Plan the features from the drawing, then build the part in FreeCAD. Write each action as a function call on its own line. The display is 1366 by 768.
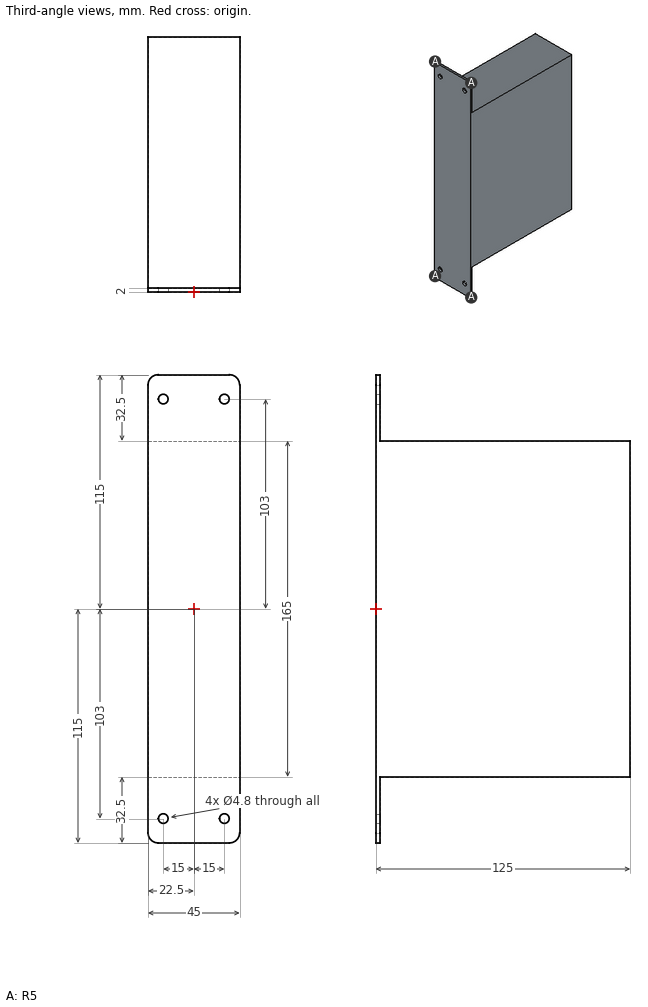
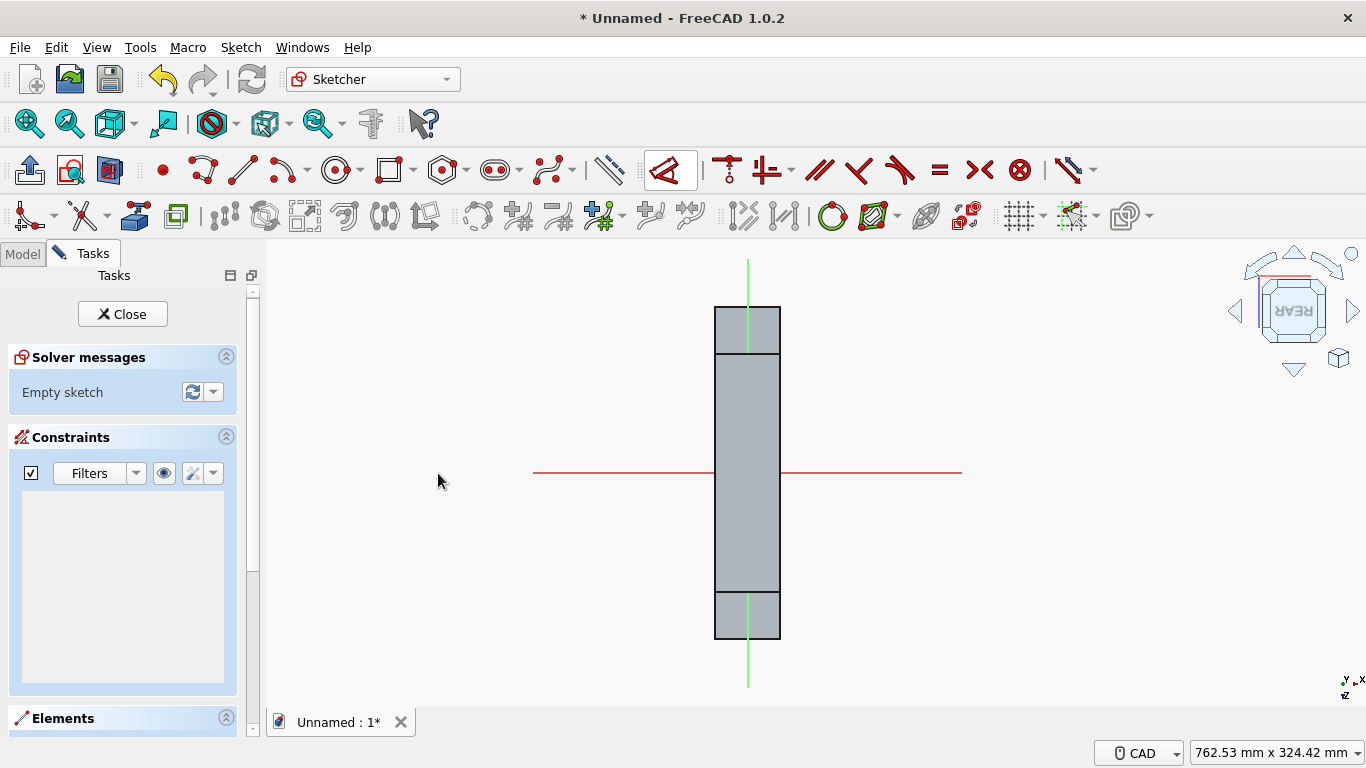
click(336, 170)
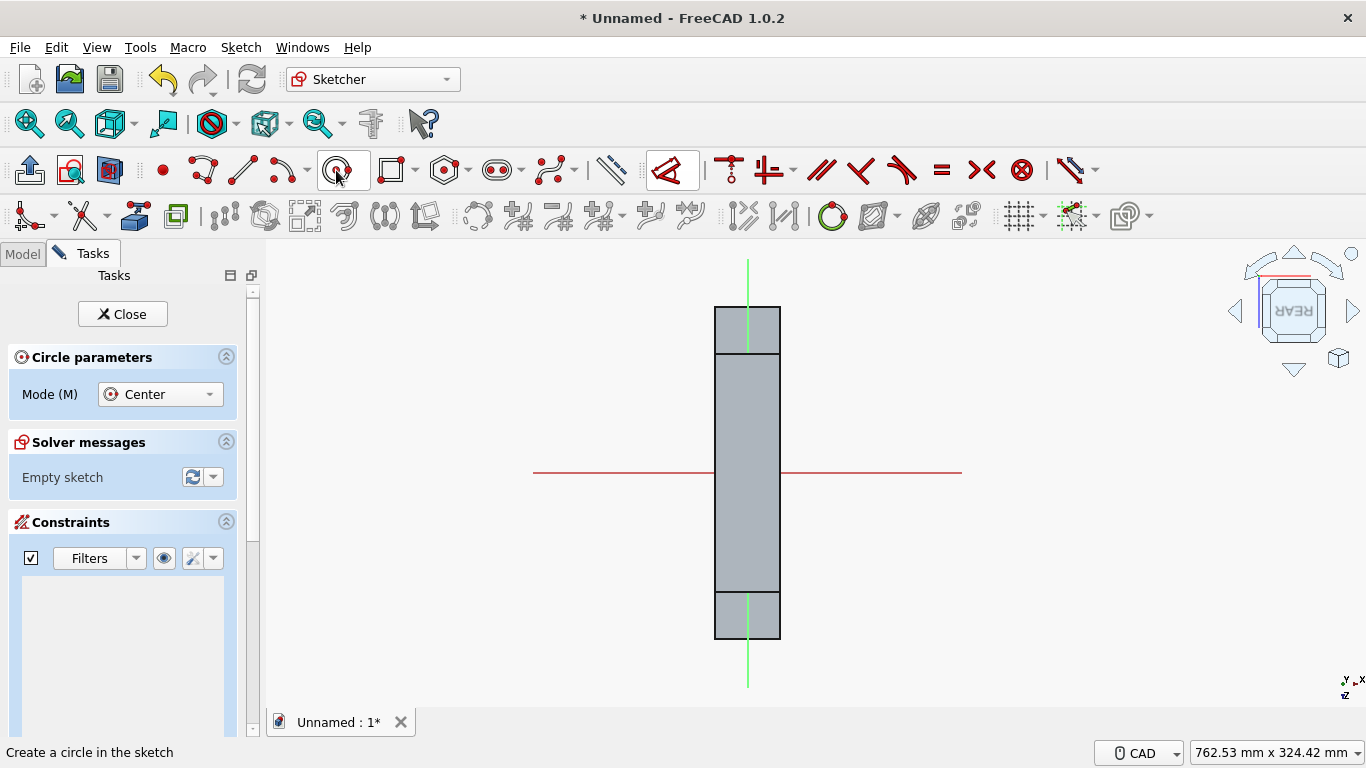
scroll(726, 325, up, 10)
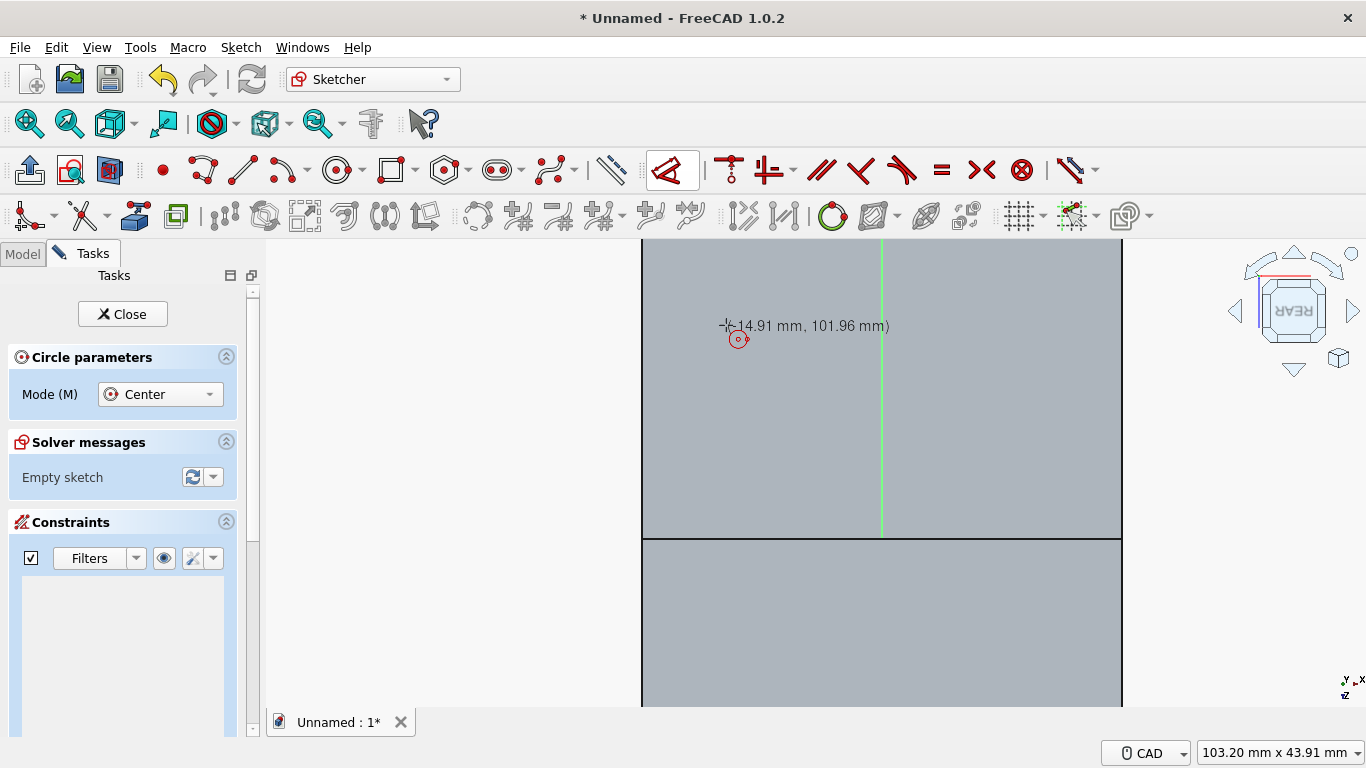
scroll(726, 325, down, 10)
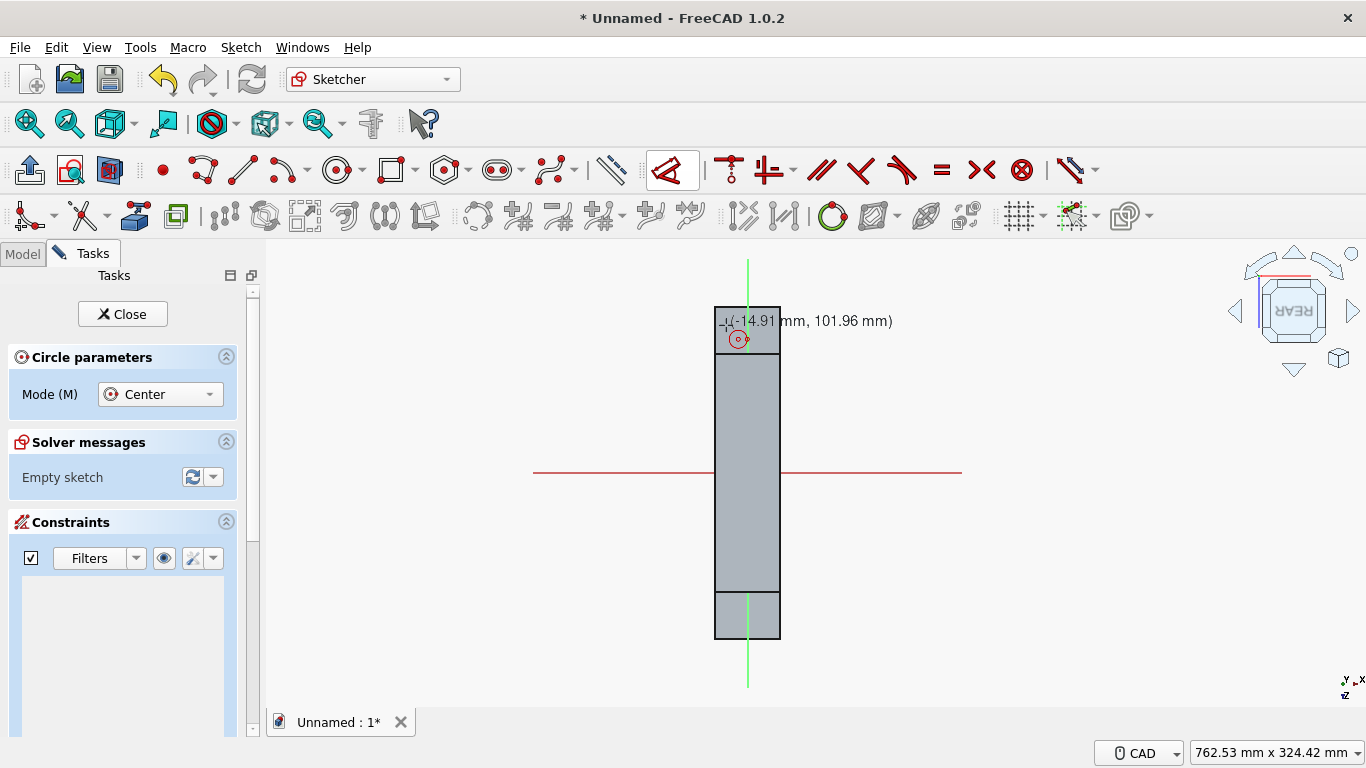
click(726, 325)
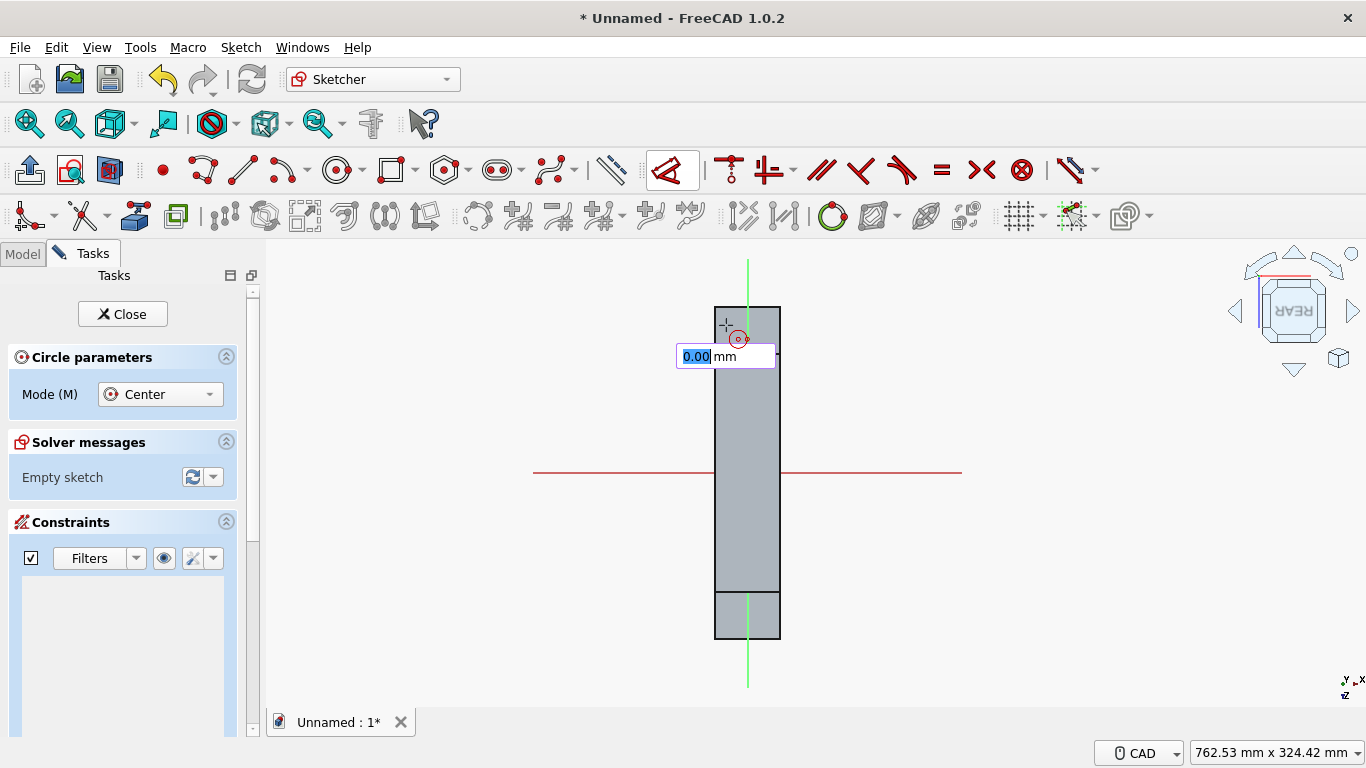
scroll(728, 322, up, 8)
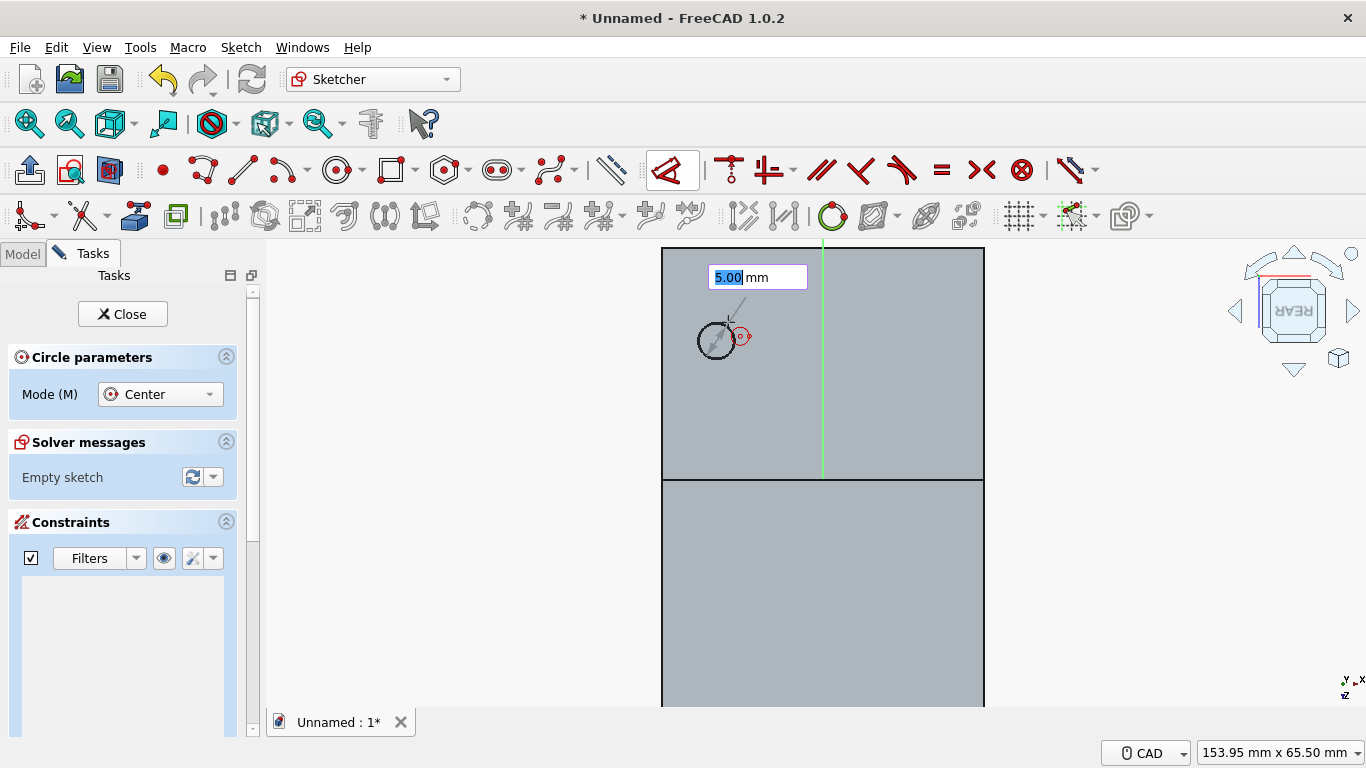
click(728, 322)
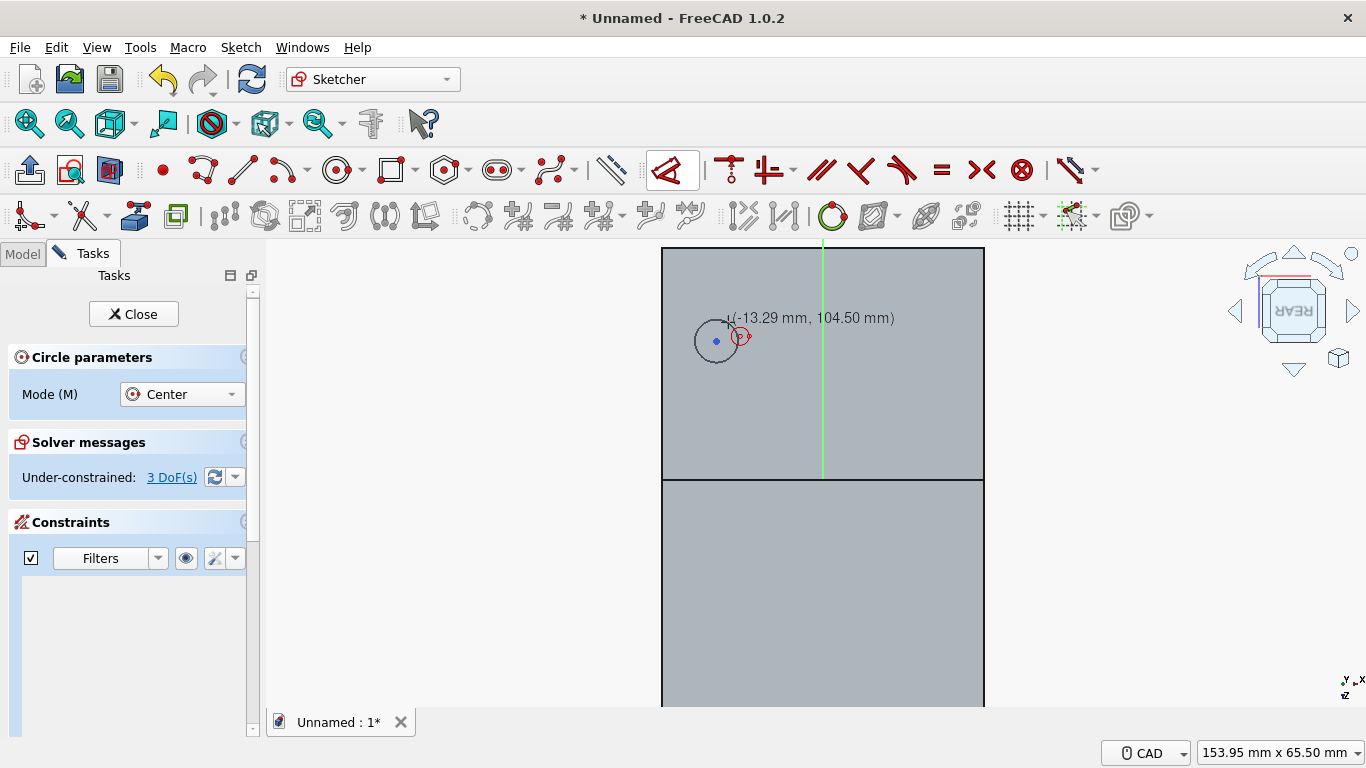
scroll(930, 334, up, 2)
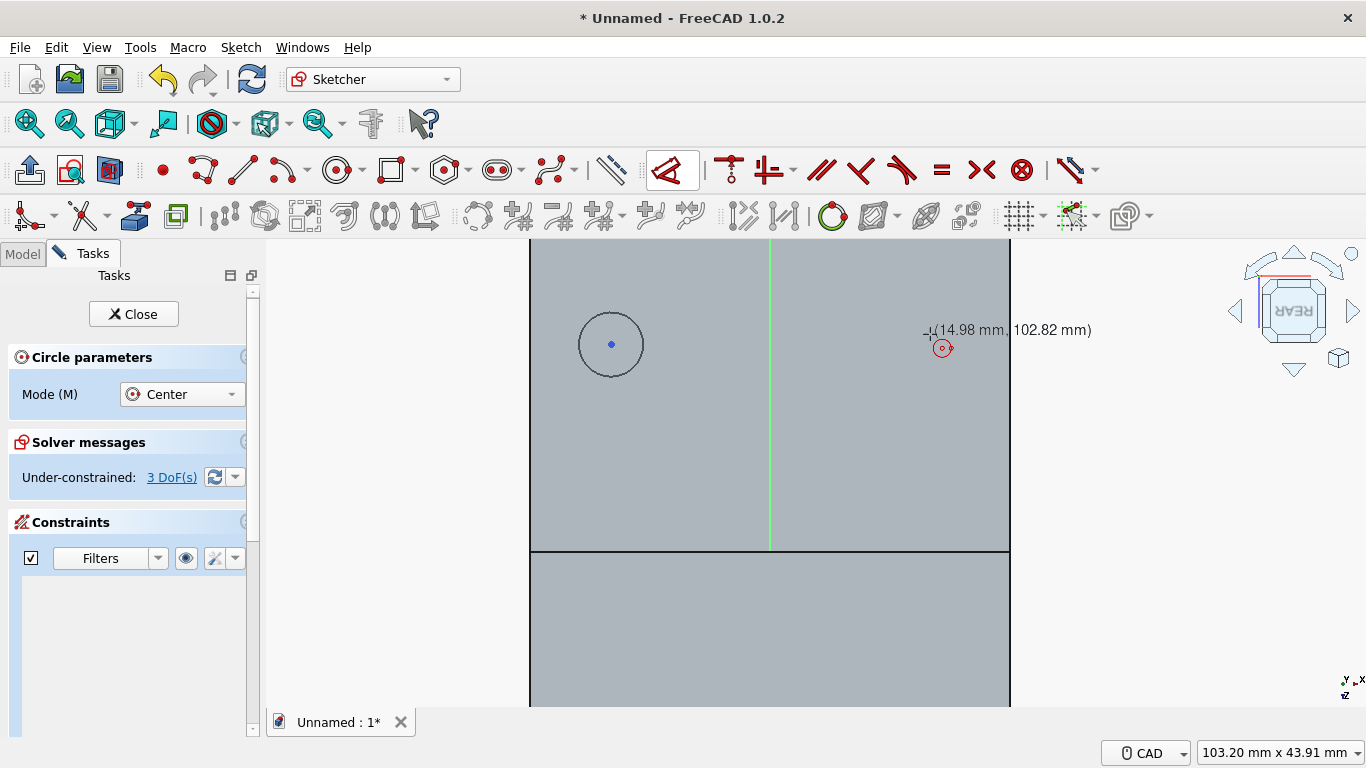
scroll(744, 323, down, 10)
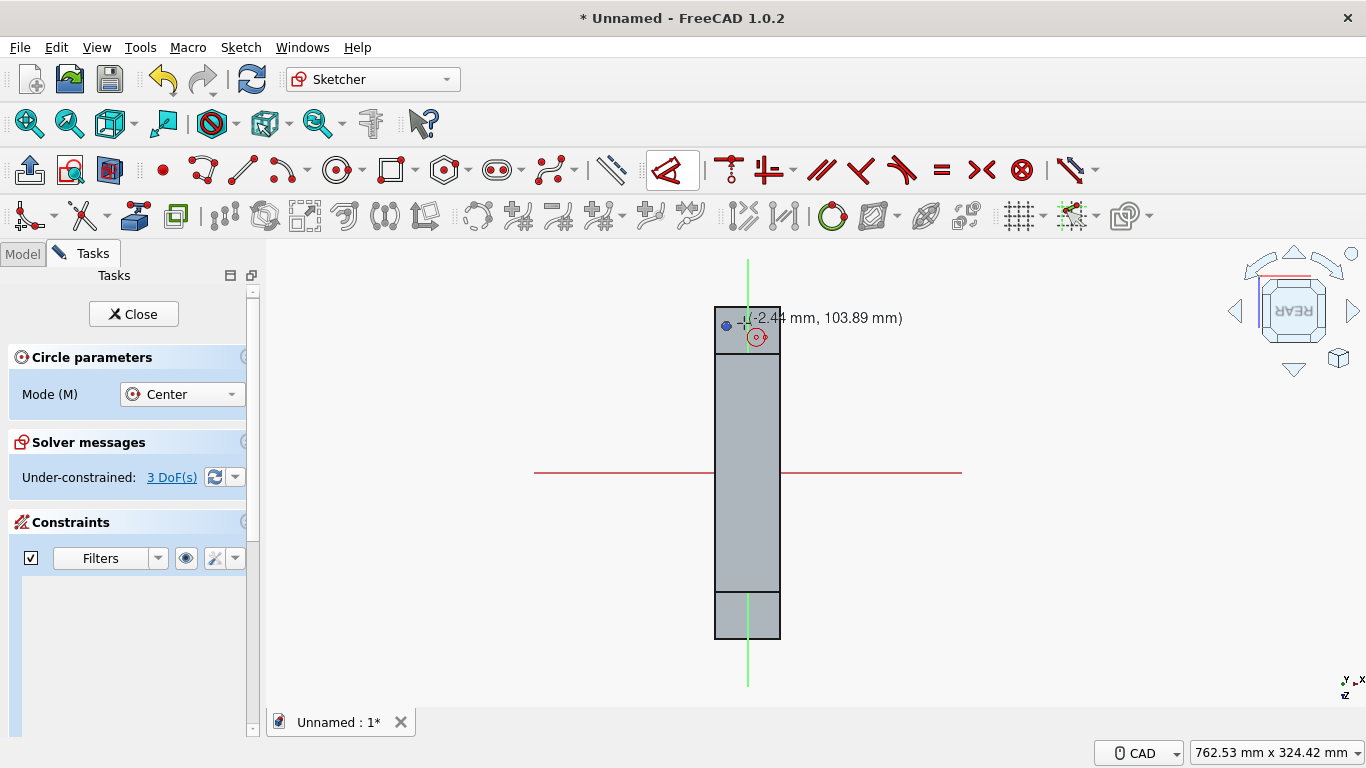
click(770, 325)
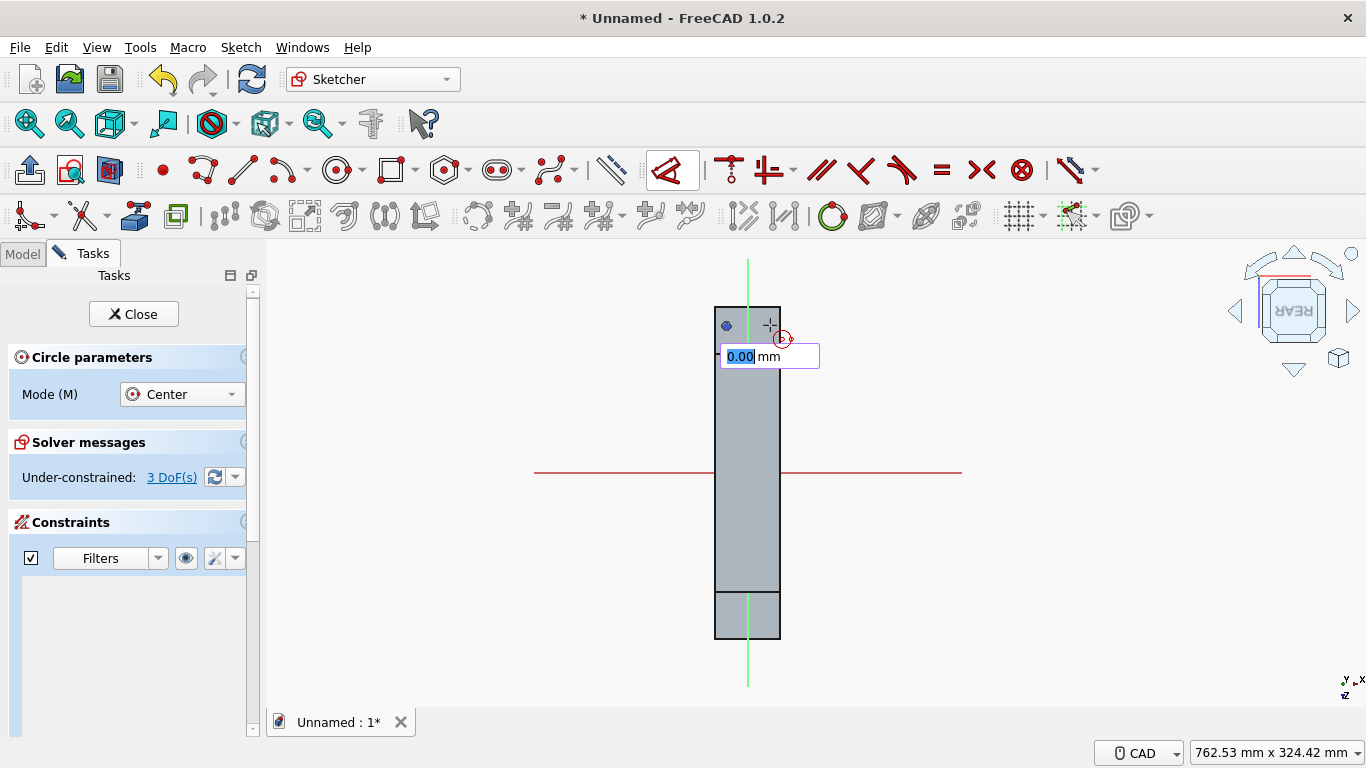
scroll(772, 322, up, 8)